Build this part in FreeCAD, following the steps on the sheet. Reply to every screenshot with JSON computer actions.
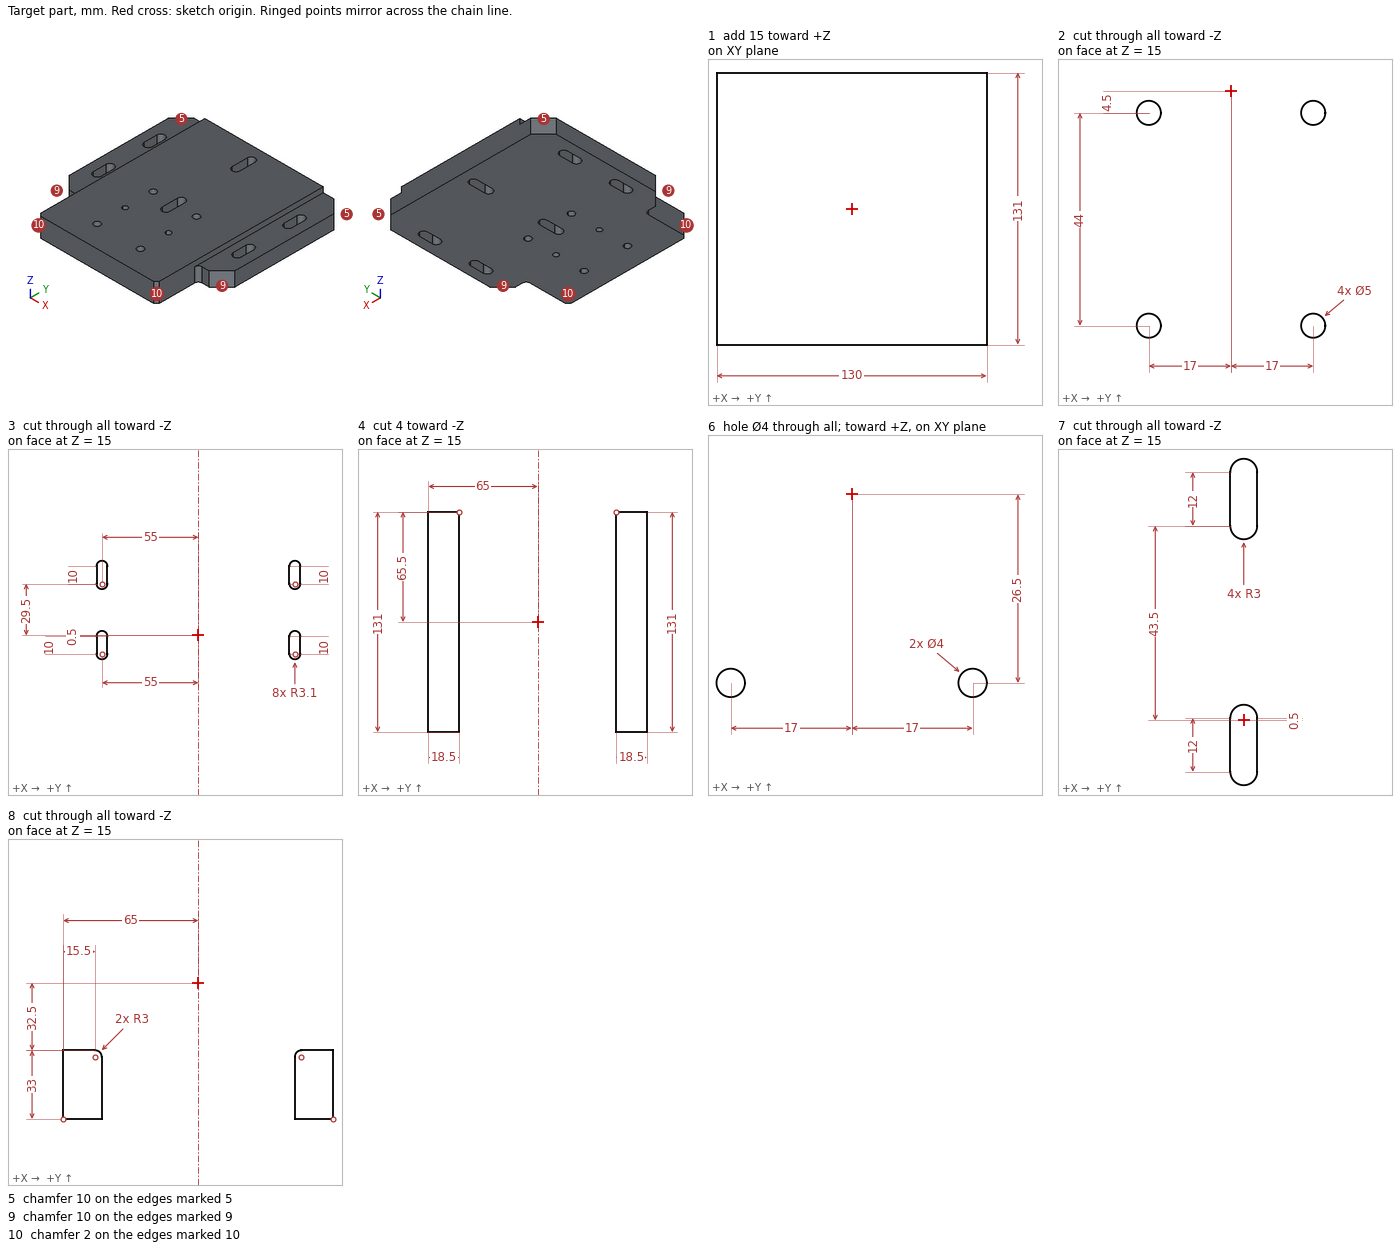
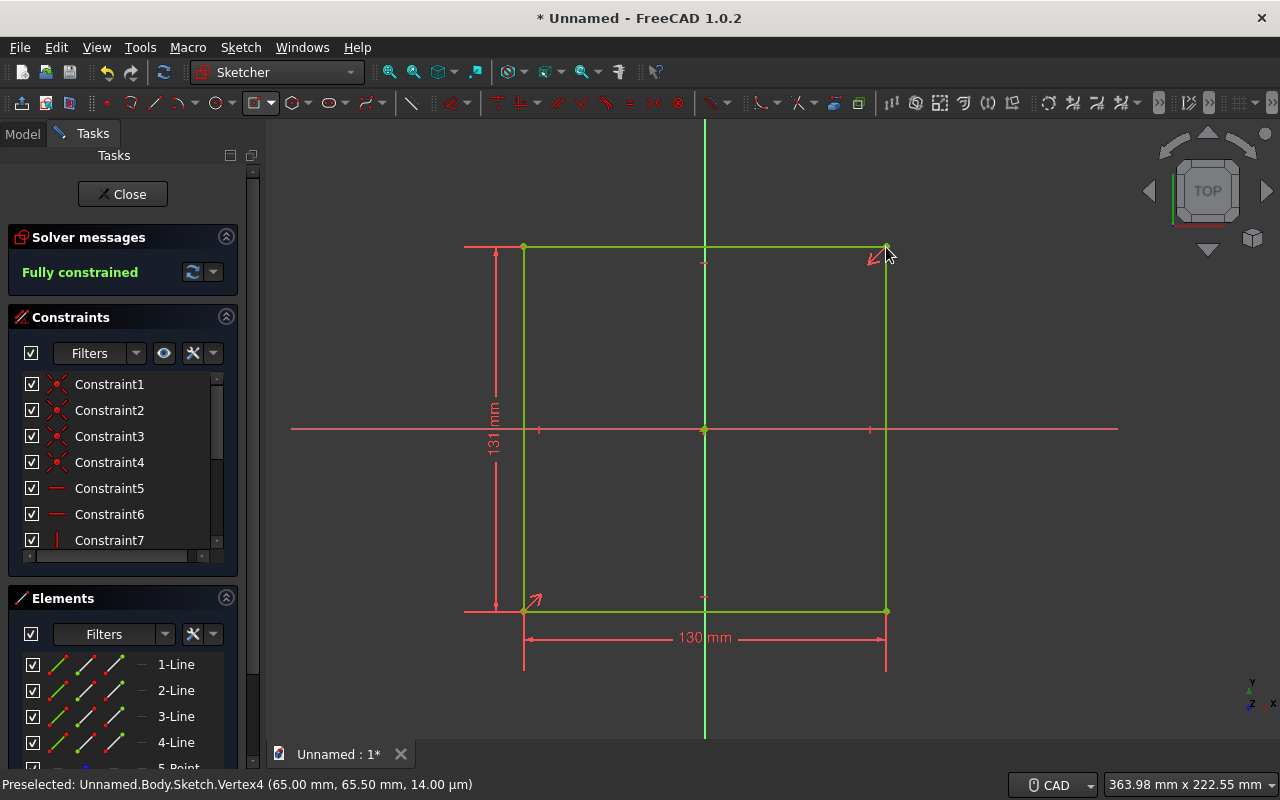
{"action": "left_click", "coordinate": [123, 194]}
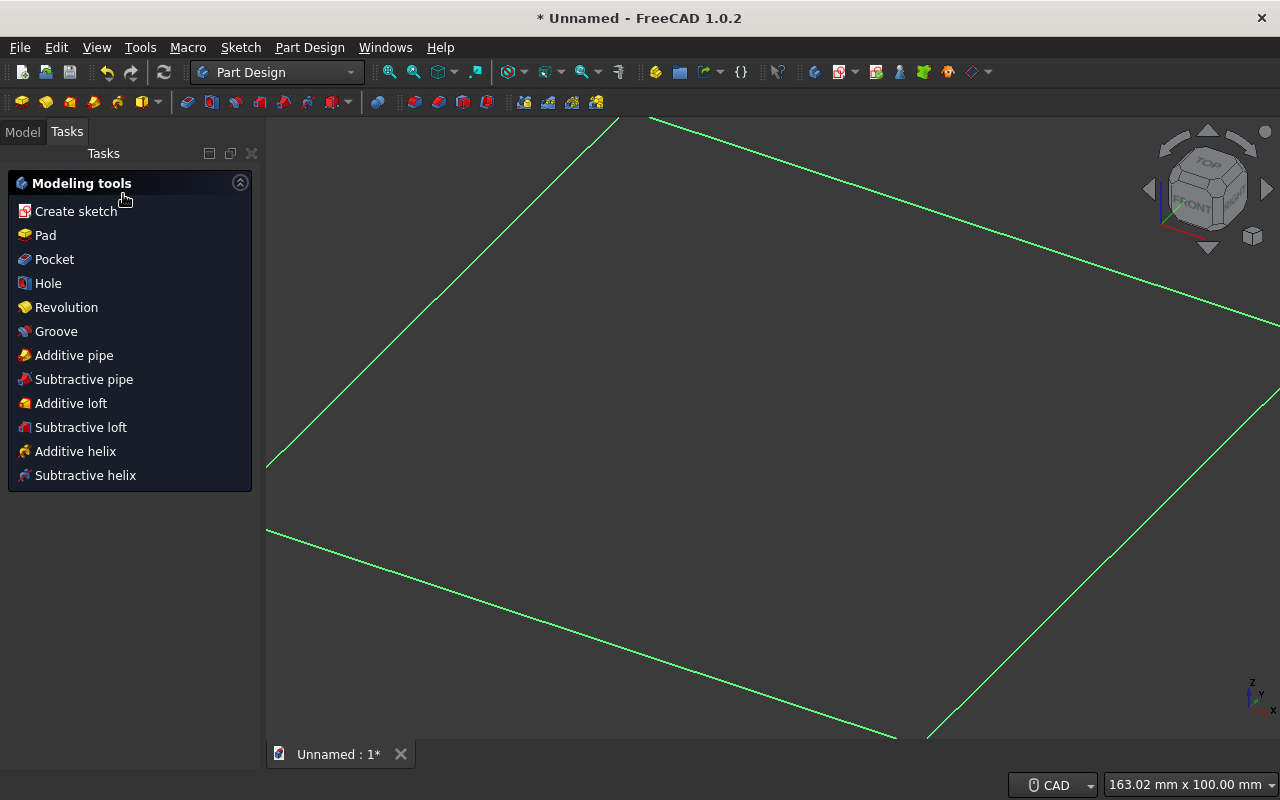
{"action": "left_click", "coordinate": [22, 102]}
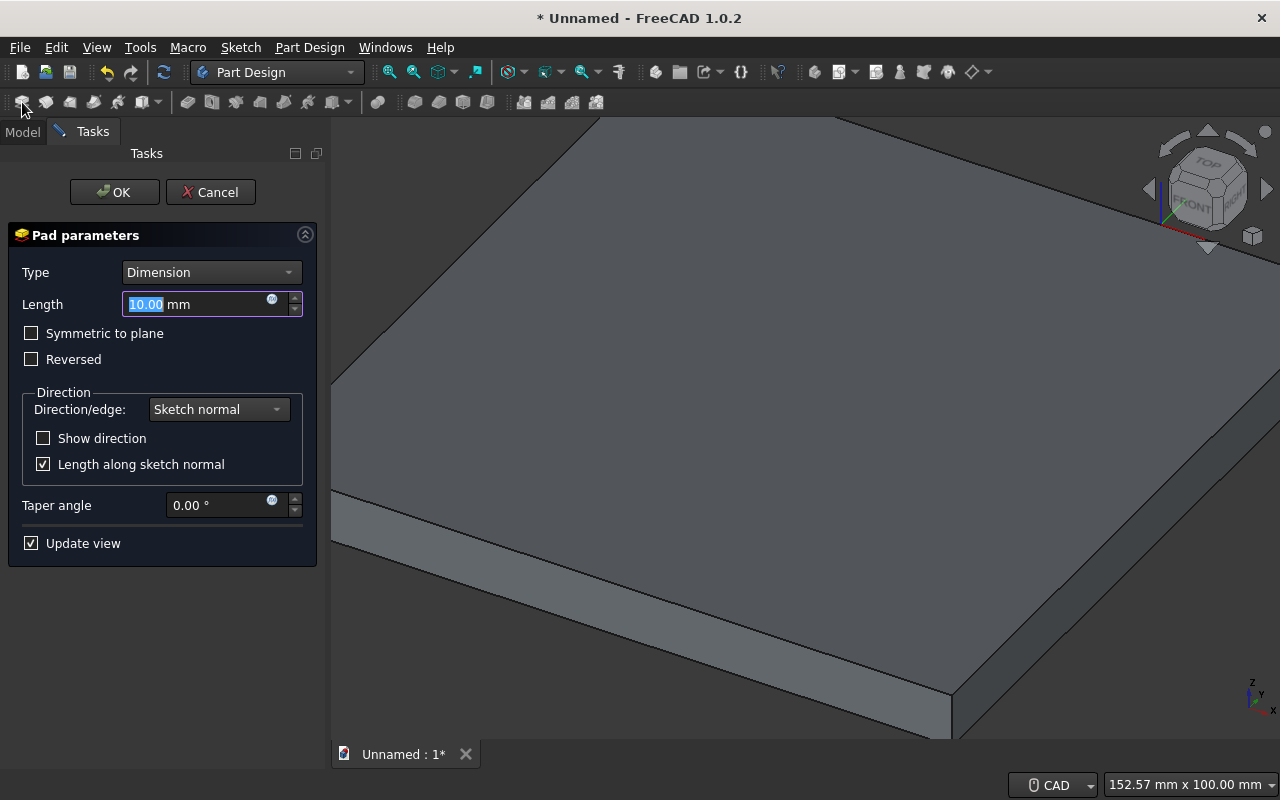
{"action": "type", "text": "15"}
{"action": "key", "text": "Tab"}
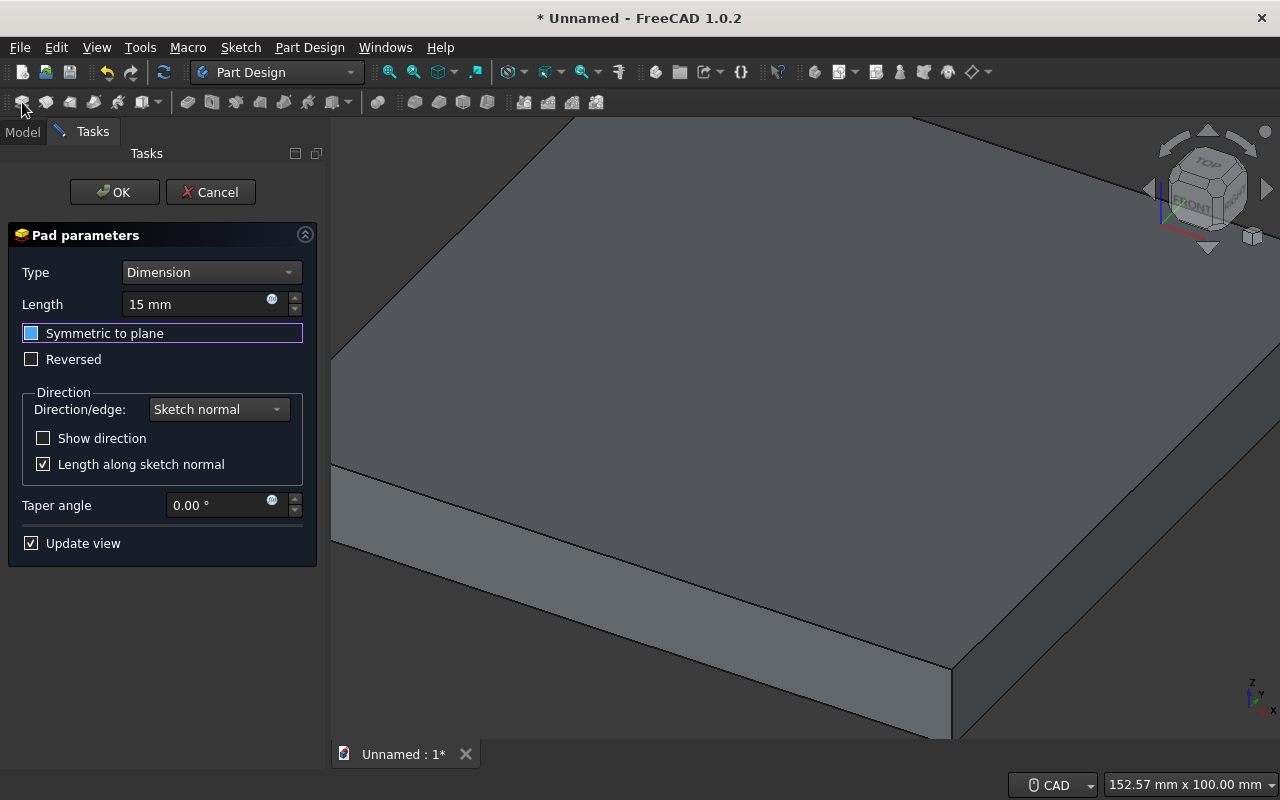
{"action": "left_click", "coordinate": [115, 192]}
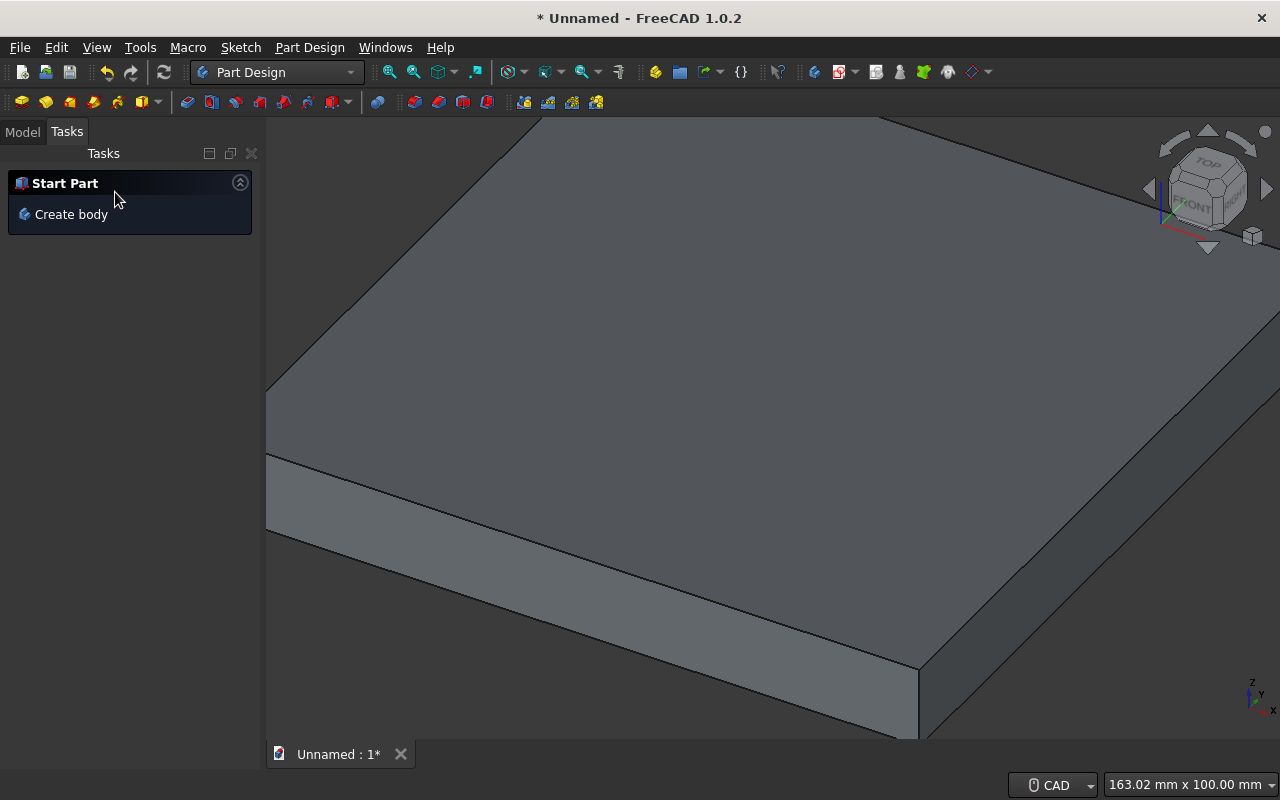
{"action": "key", "text": "v f"}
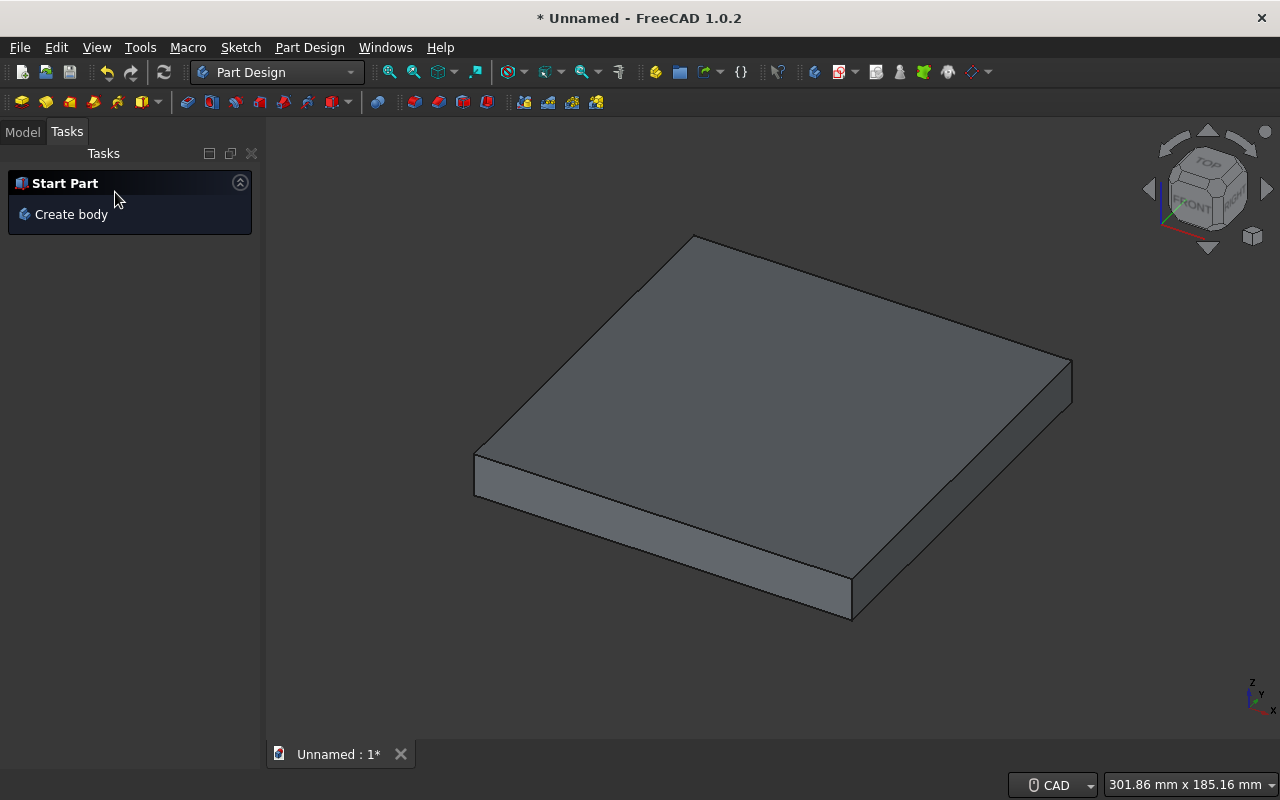
{"action": "left_click", "coordinate": [773, 406]}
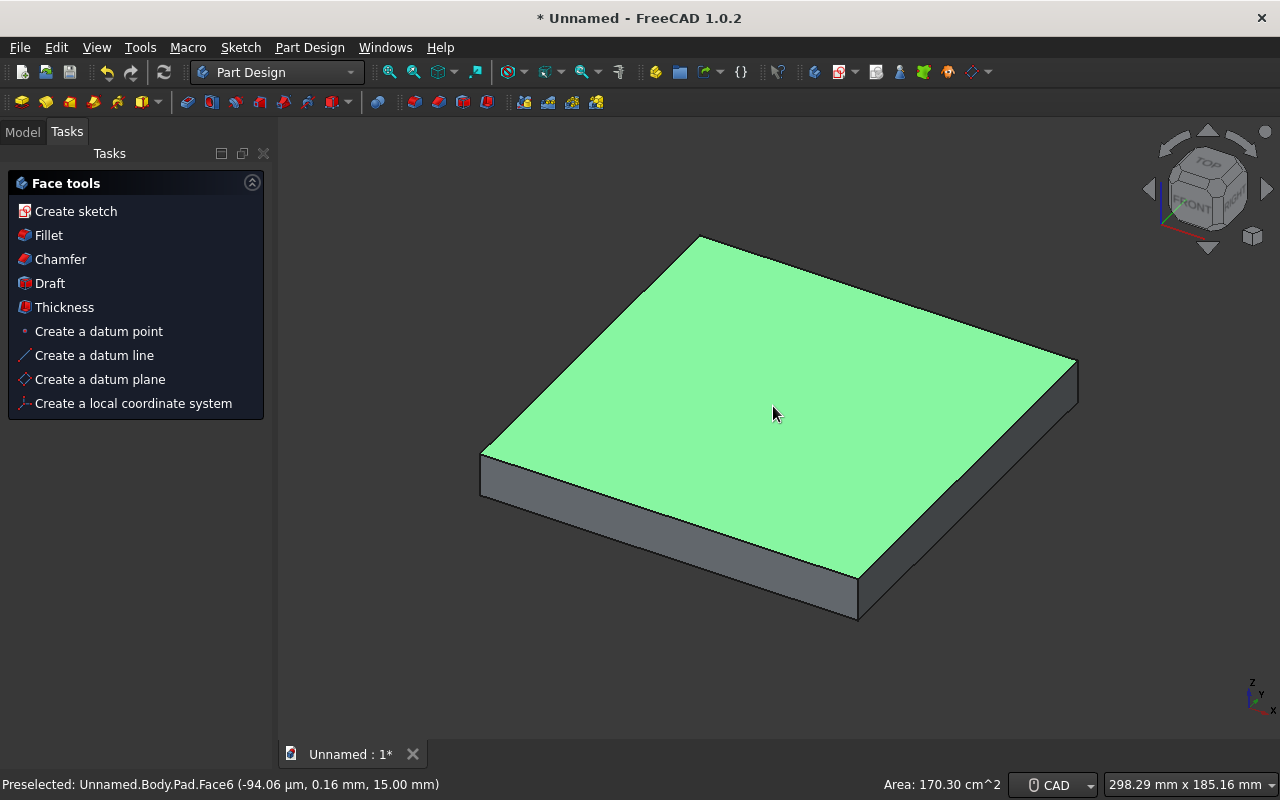
{"action": "left_click", "coordinate": [840, 72]}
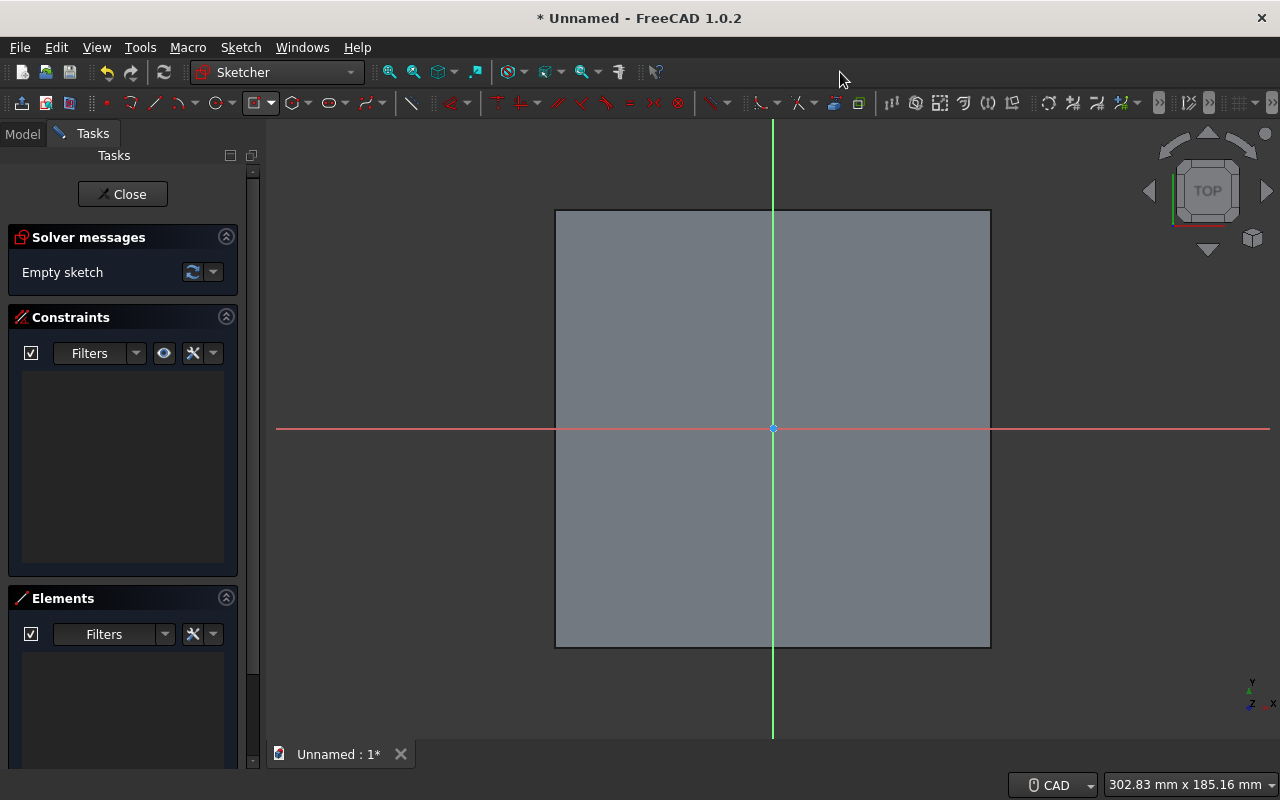
{"action": "scroll", "coordinate": [829, 584], "scroll_direction": "up", "scroll_amount": 4}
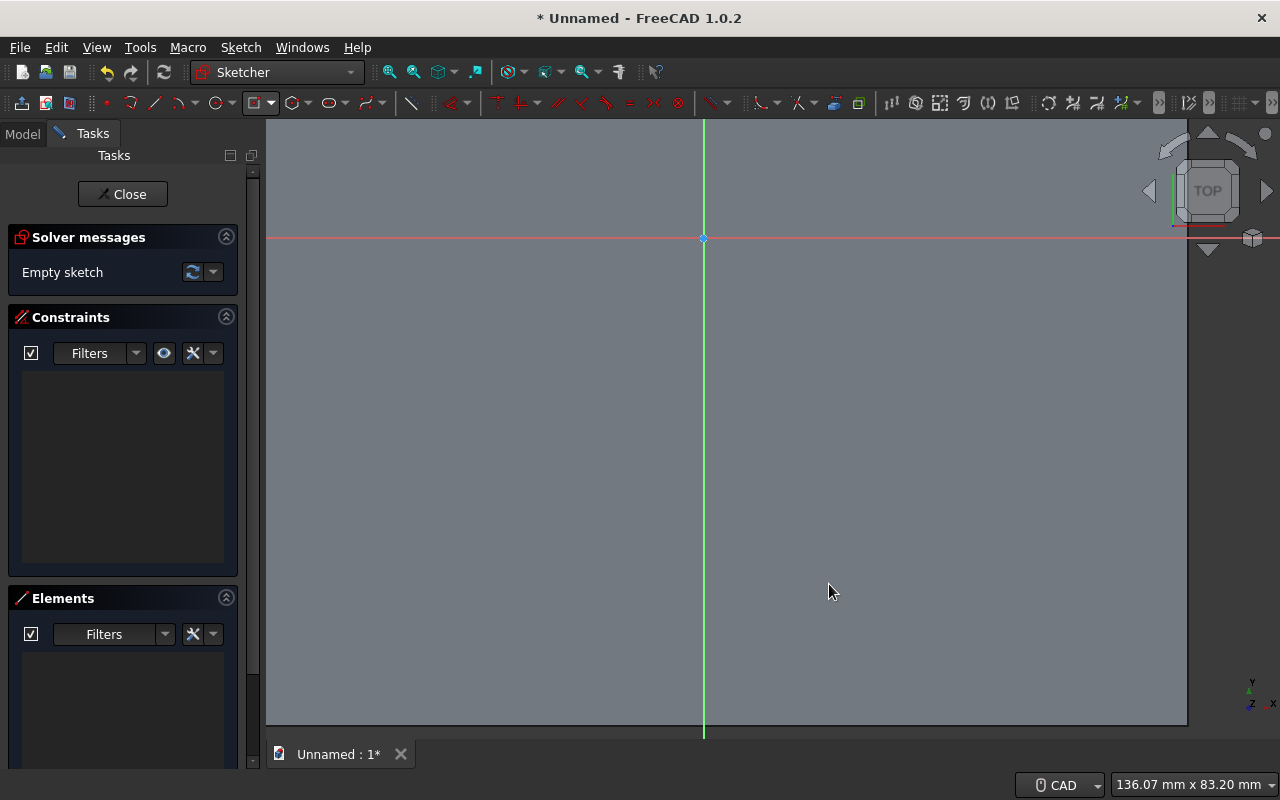
{"action": "key", "text": "g c"}